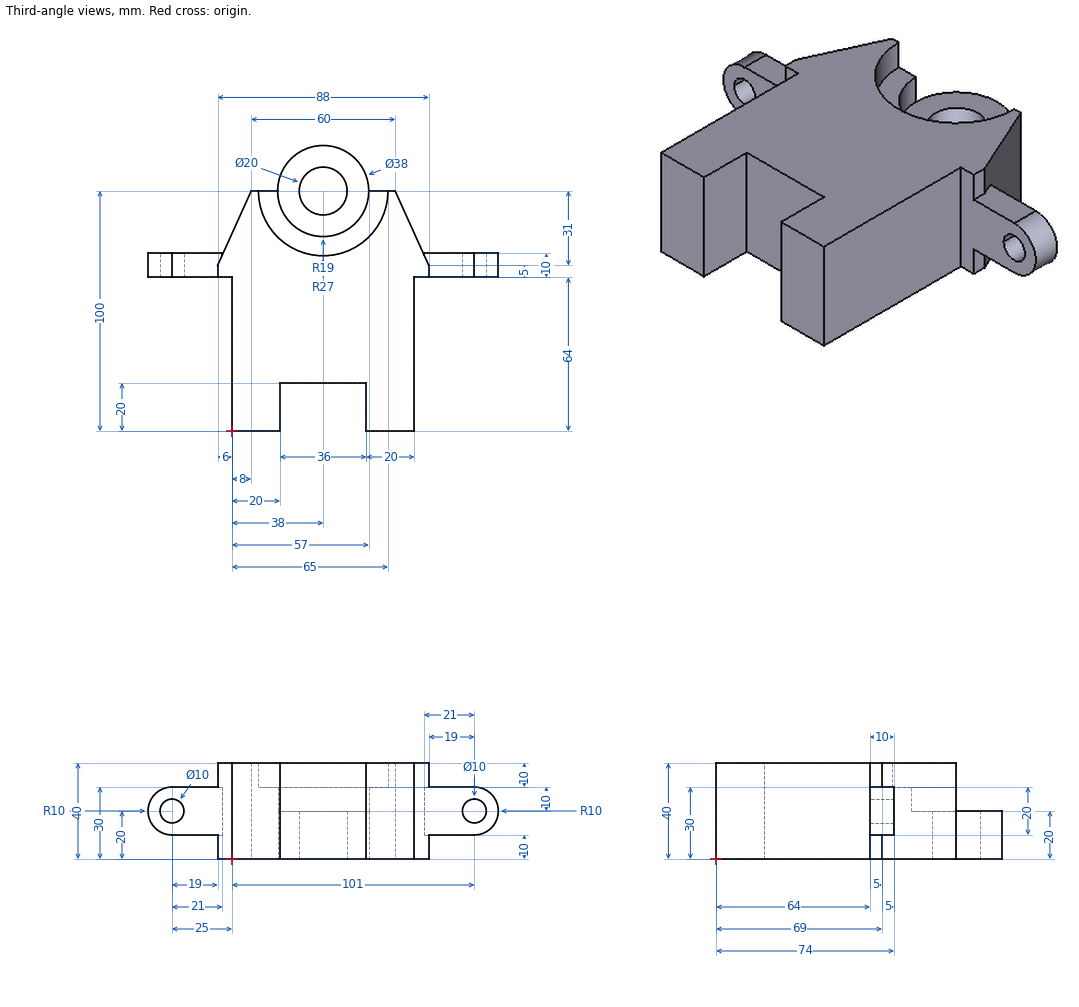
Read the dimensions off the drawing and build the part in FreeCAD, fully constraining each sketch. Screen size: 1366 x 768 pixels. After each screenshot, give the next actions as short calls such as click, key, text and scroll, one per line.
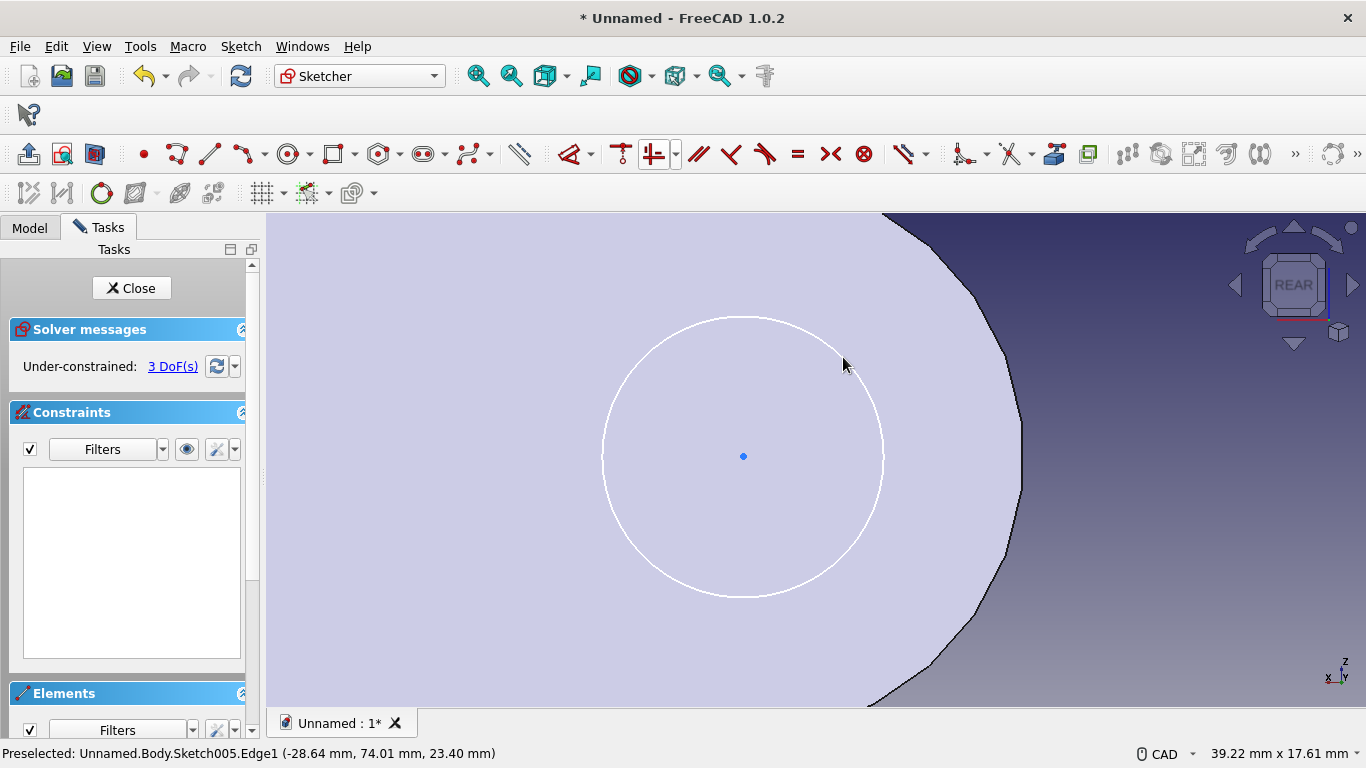
click(568, 154)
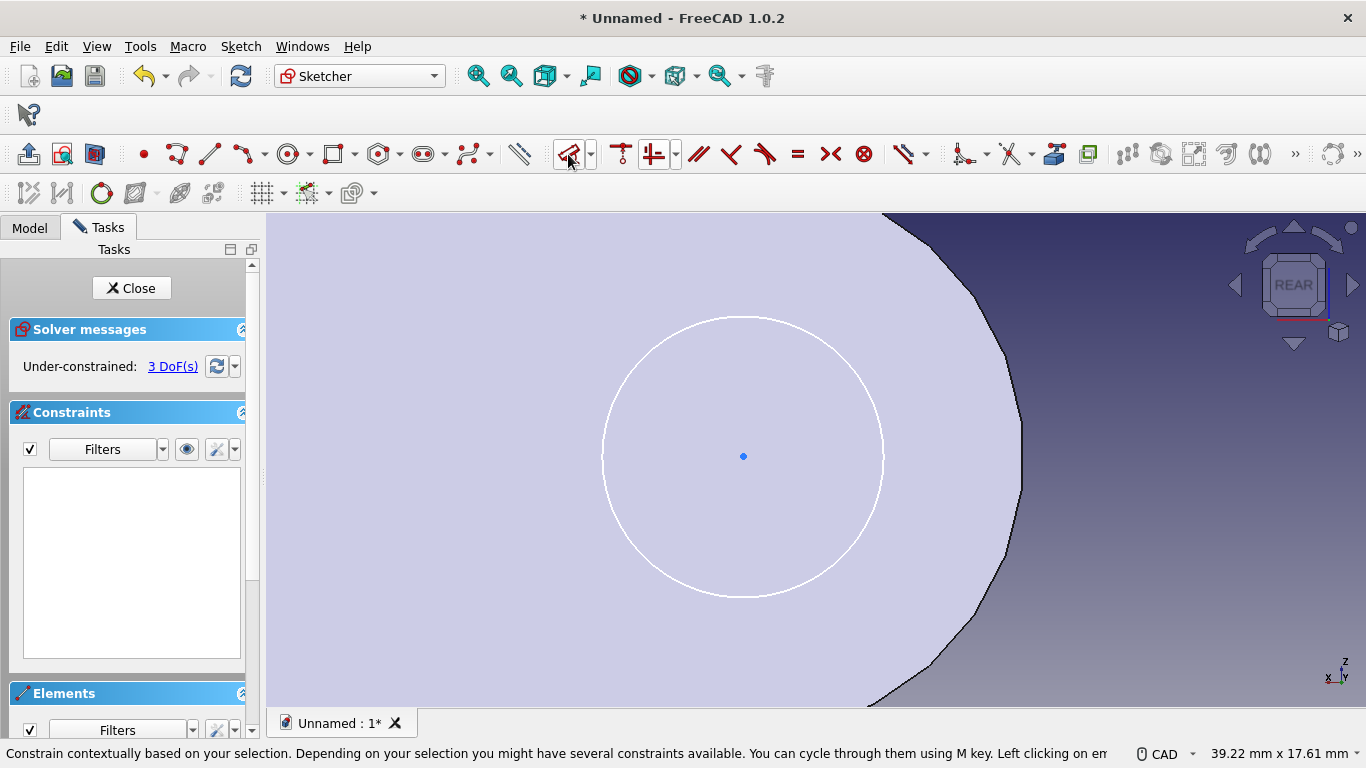
click(842, 357)
click(865, 334)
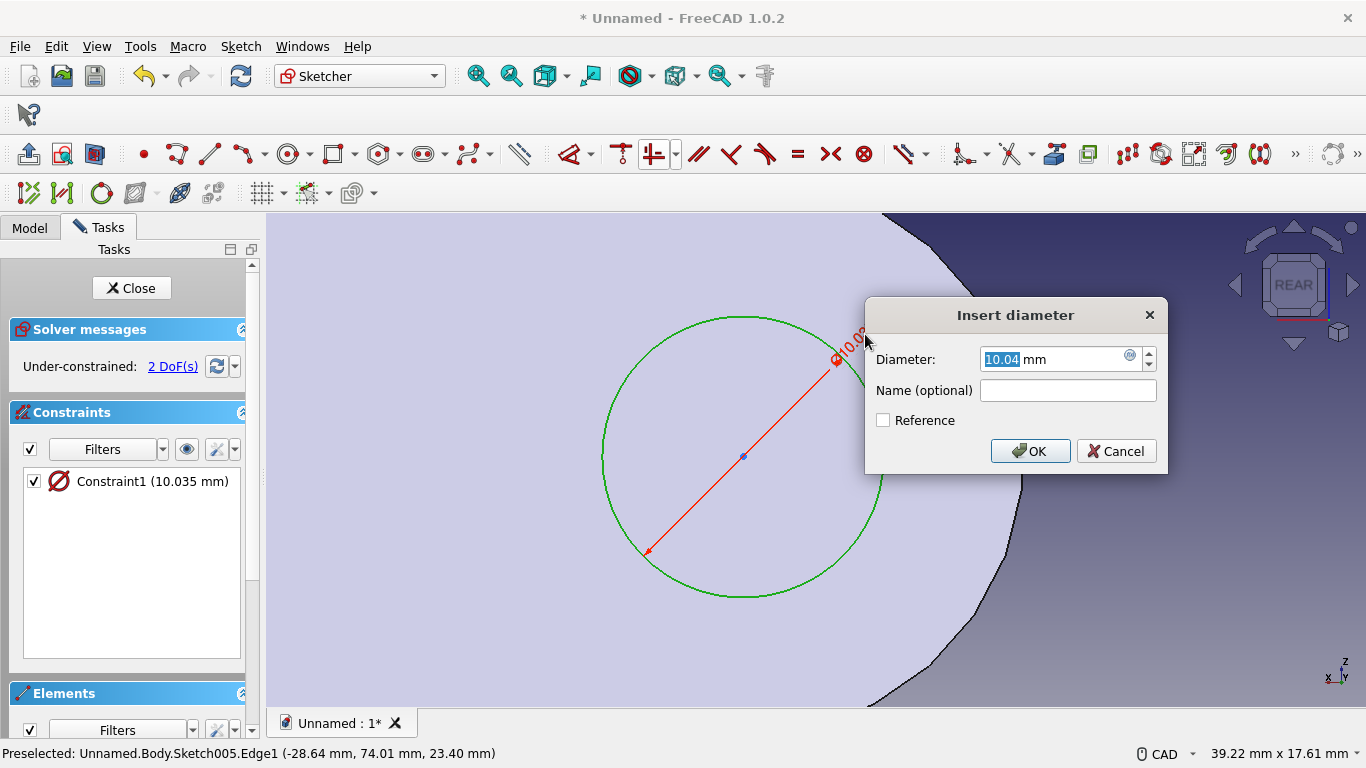
text(10)
key(Return)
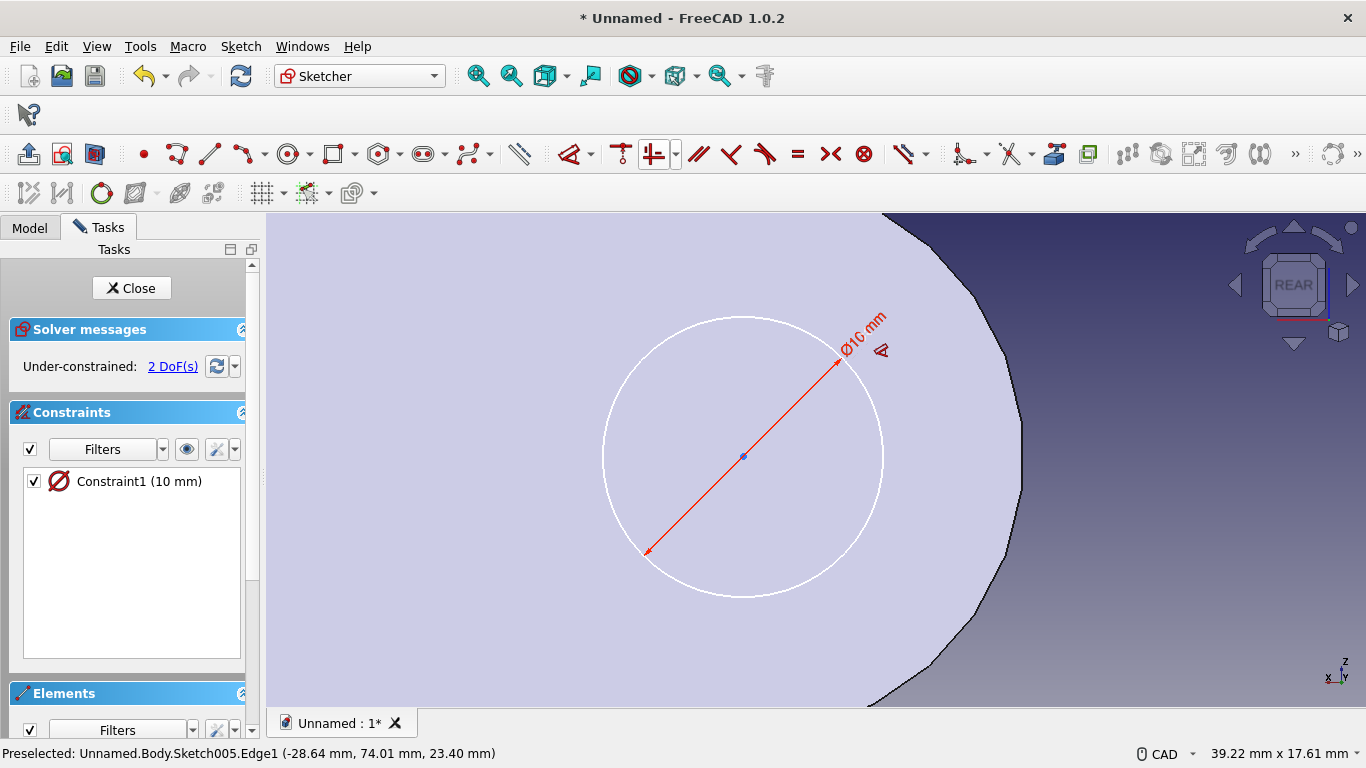
click(743, 457)
click(518, 423)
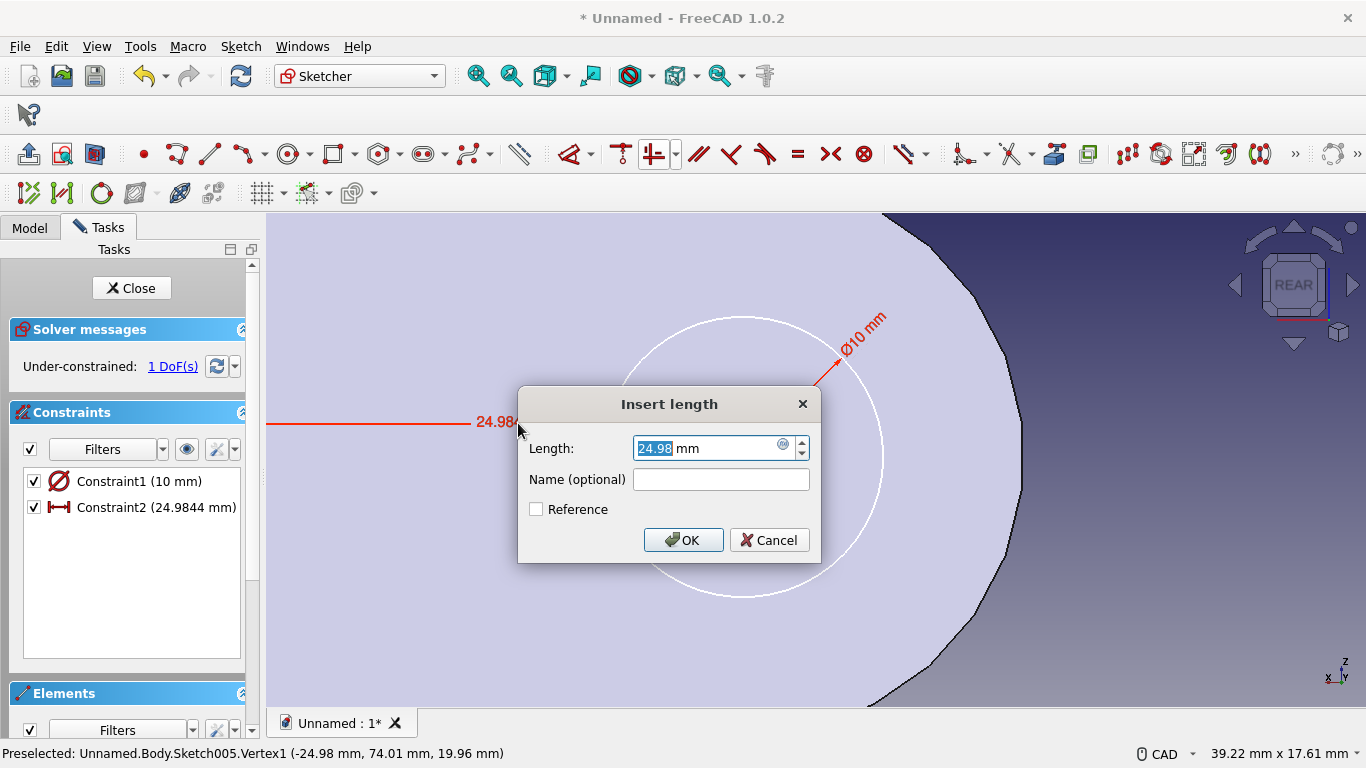
text(25)
key(Return)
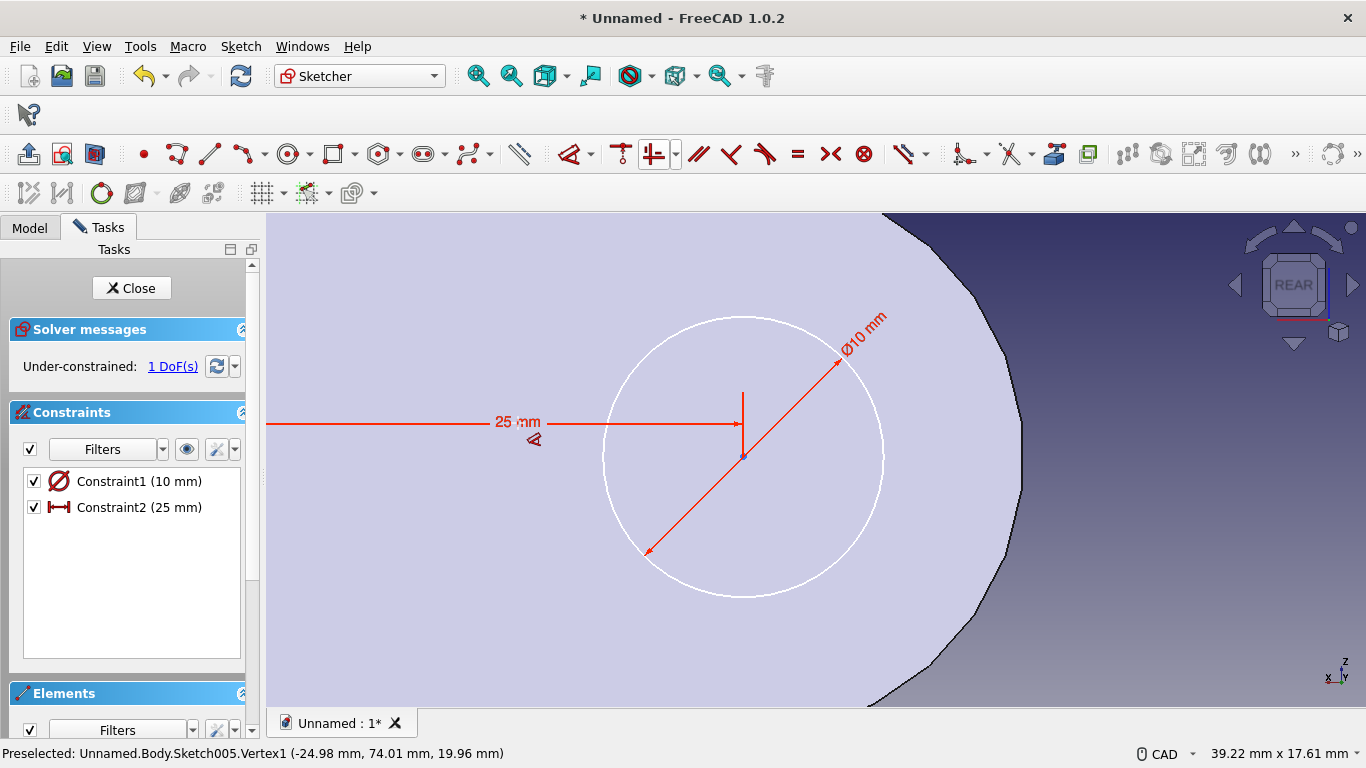
click(743, 457)
click(777, 568)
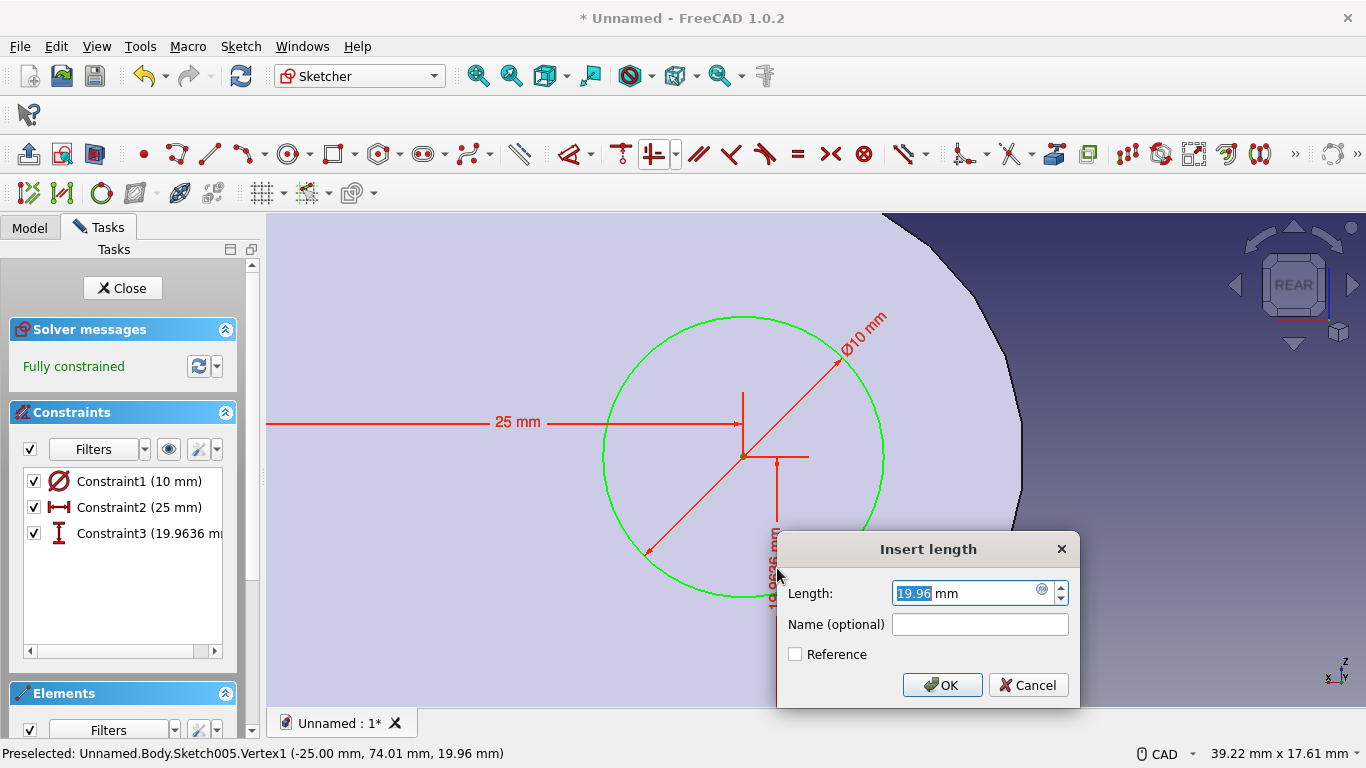
text(20)
key(Return)
key(Escape)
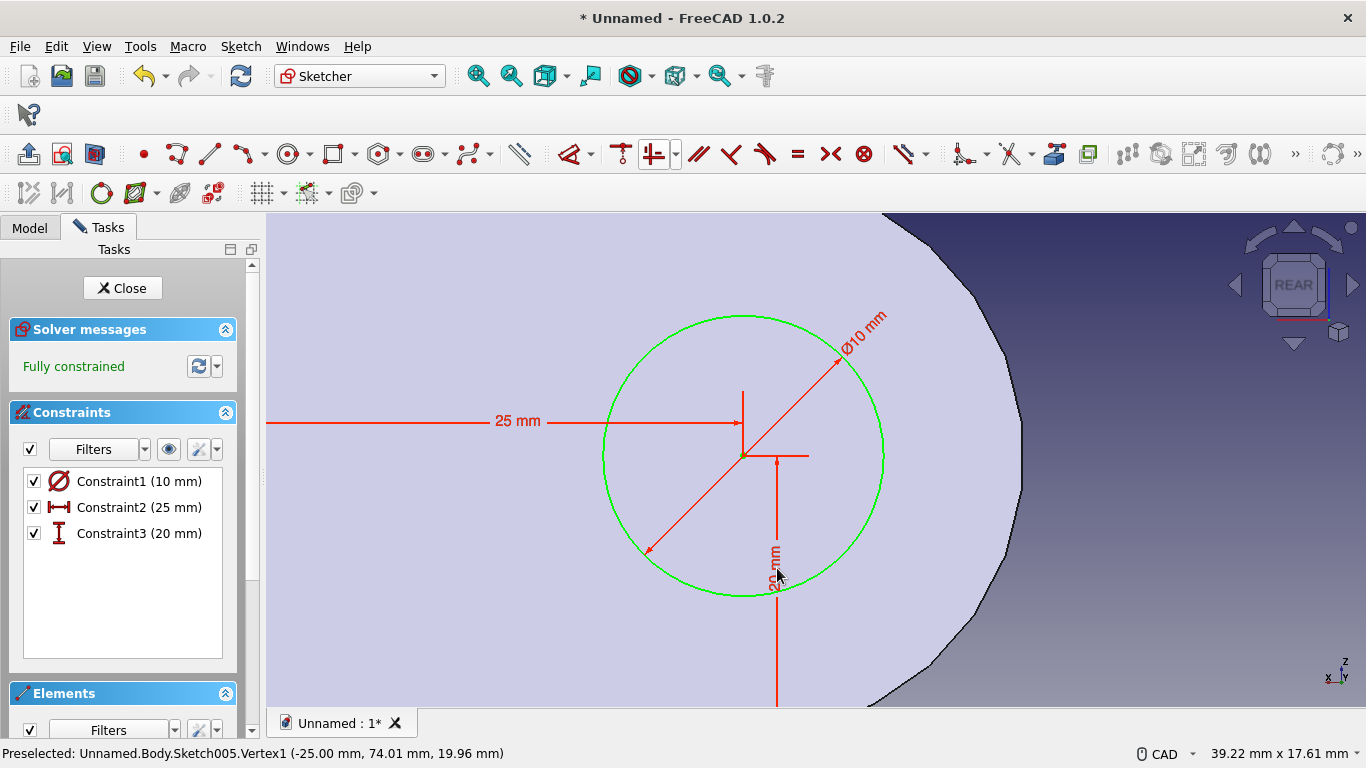
click(123, 288)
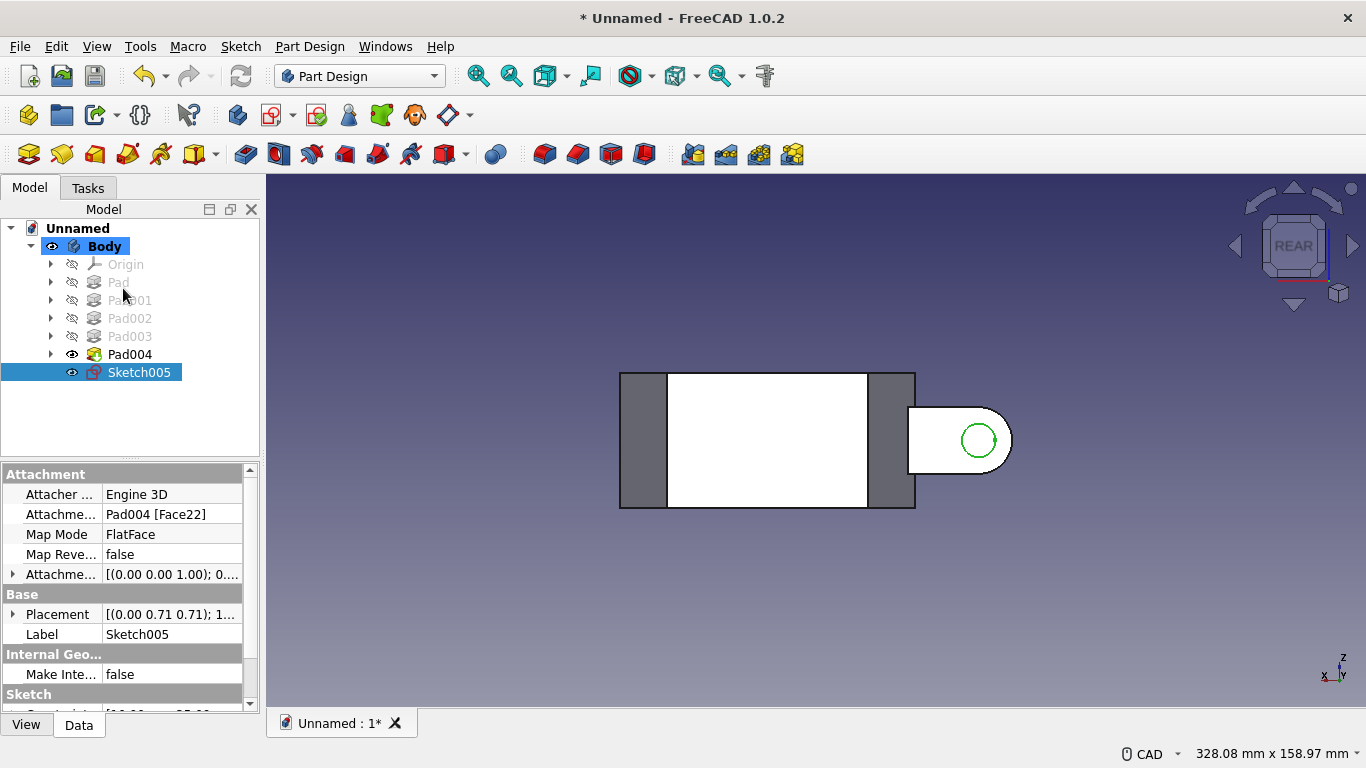
click(246, 154)